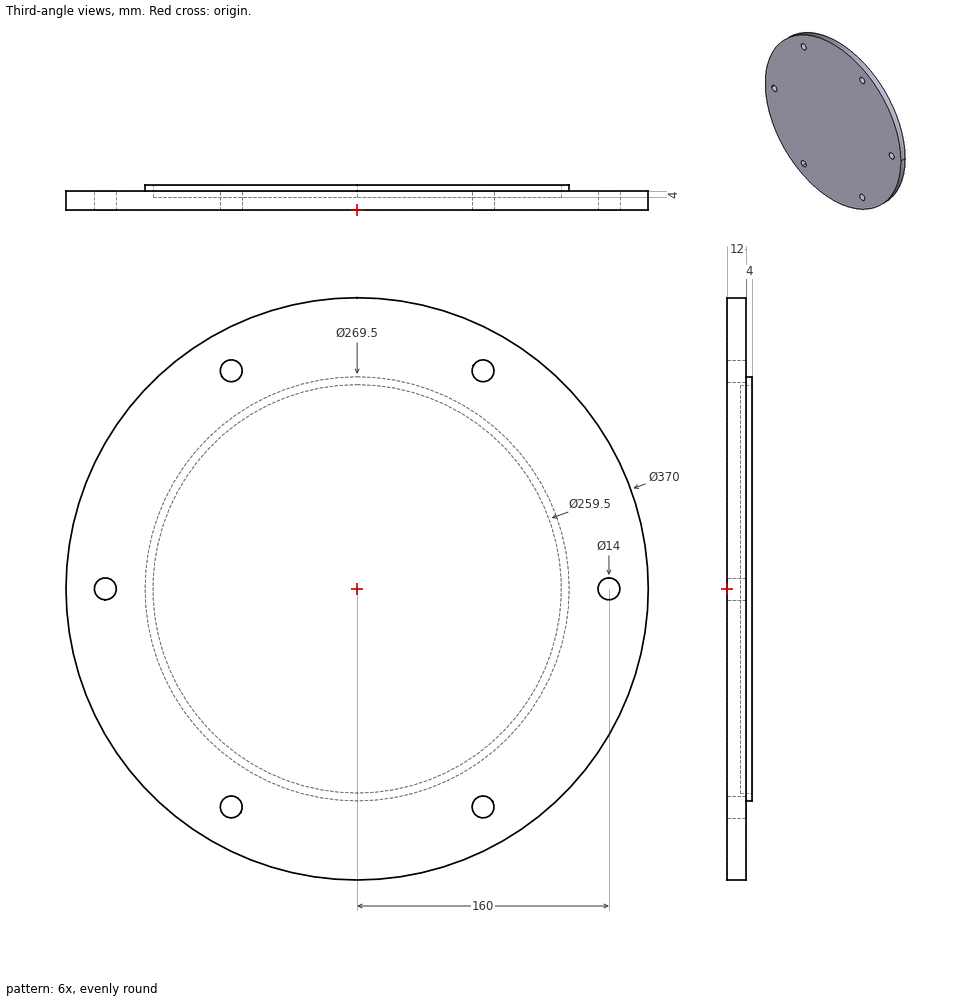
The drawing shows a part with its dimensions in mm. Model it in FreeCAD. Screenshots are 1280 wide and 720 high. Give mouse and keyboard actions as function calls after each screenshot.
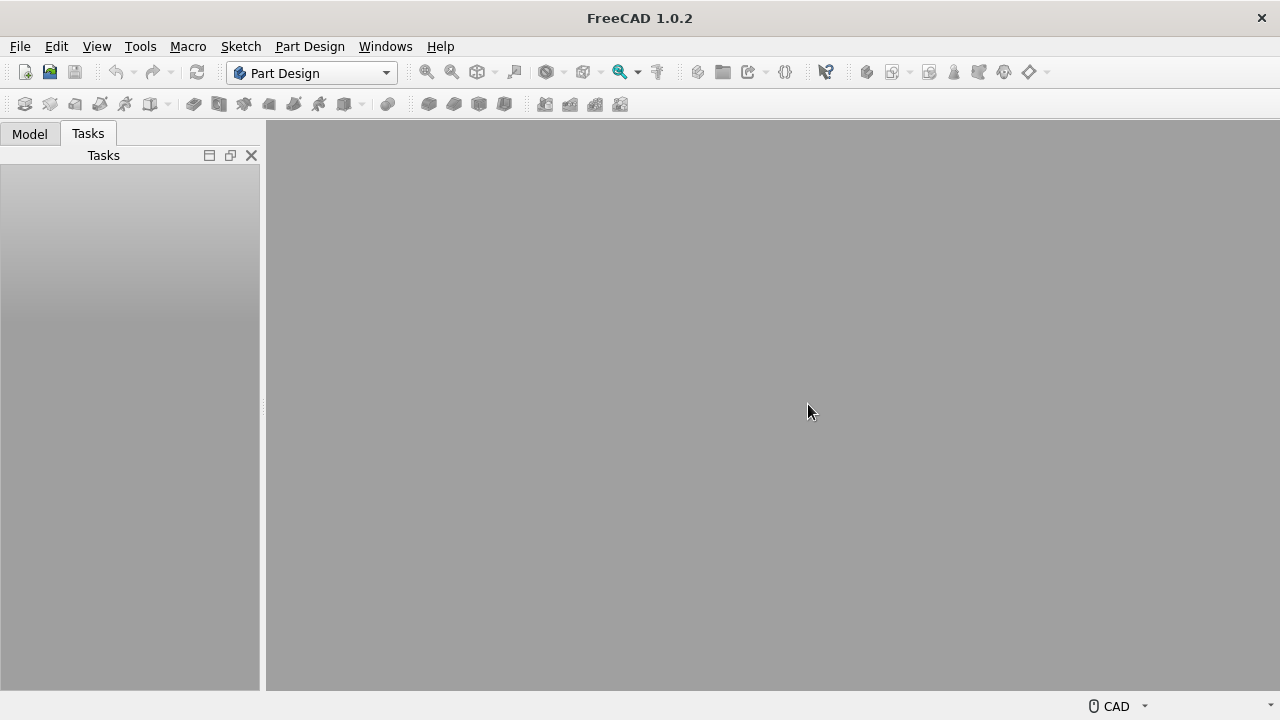
click(25, 72)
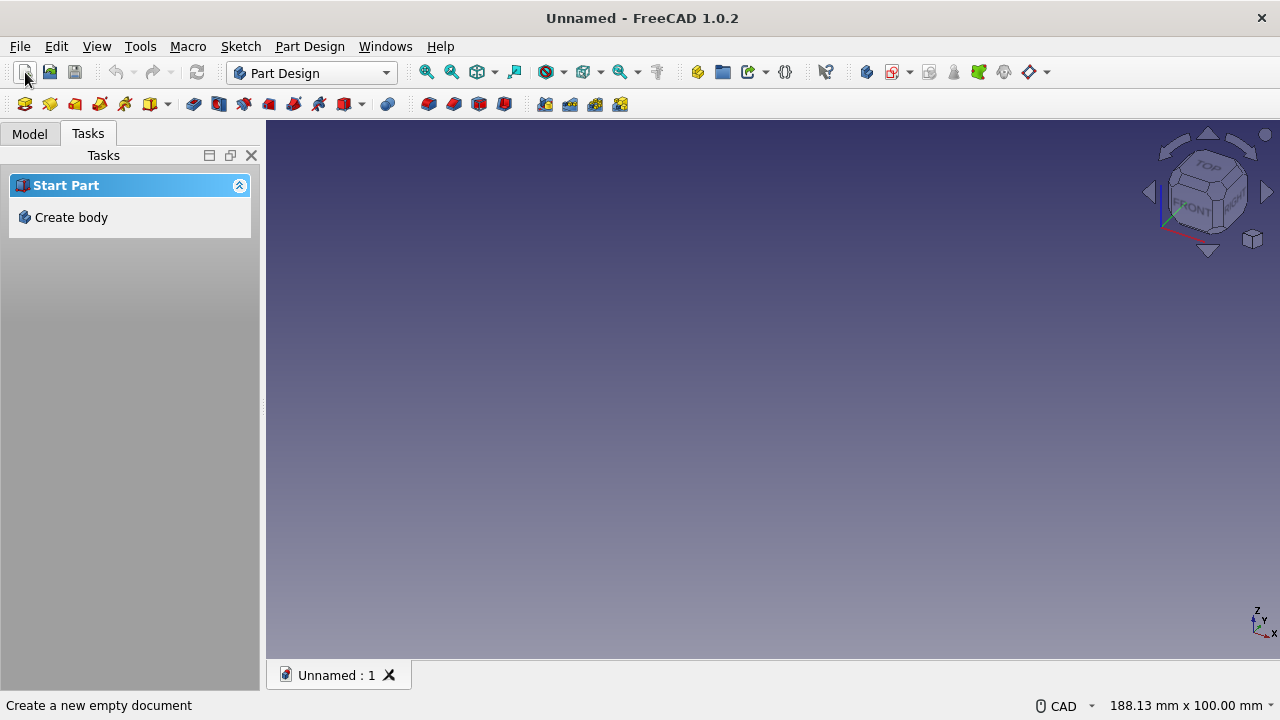
click(892, 72)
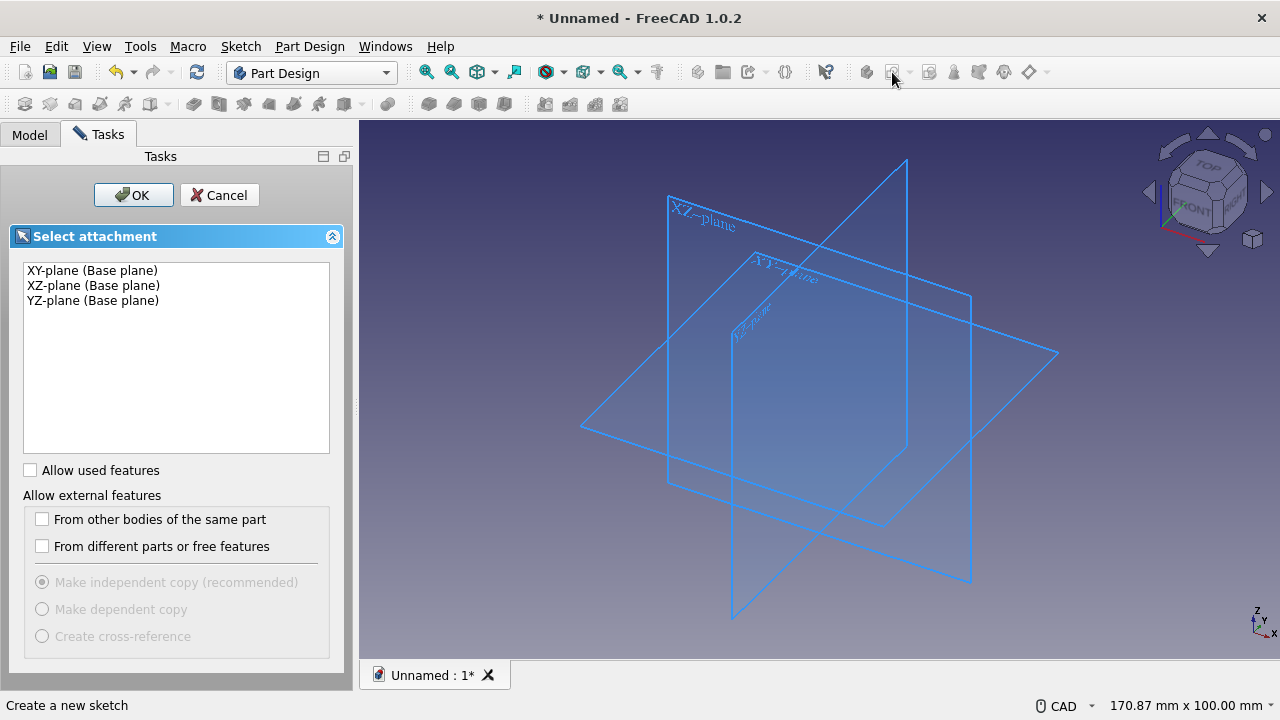
click(84, 286)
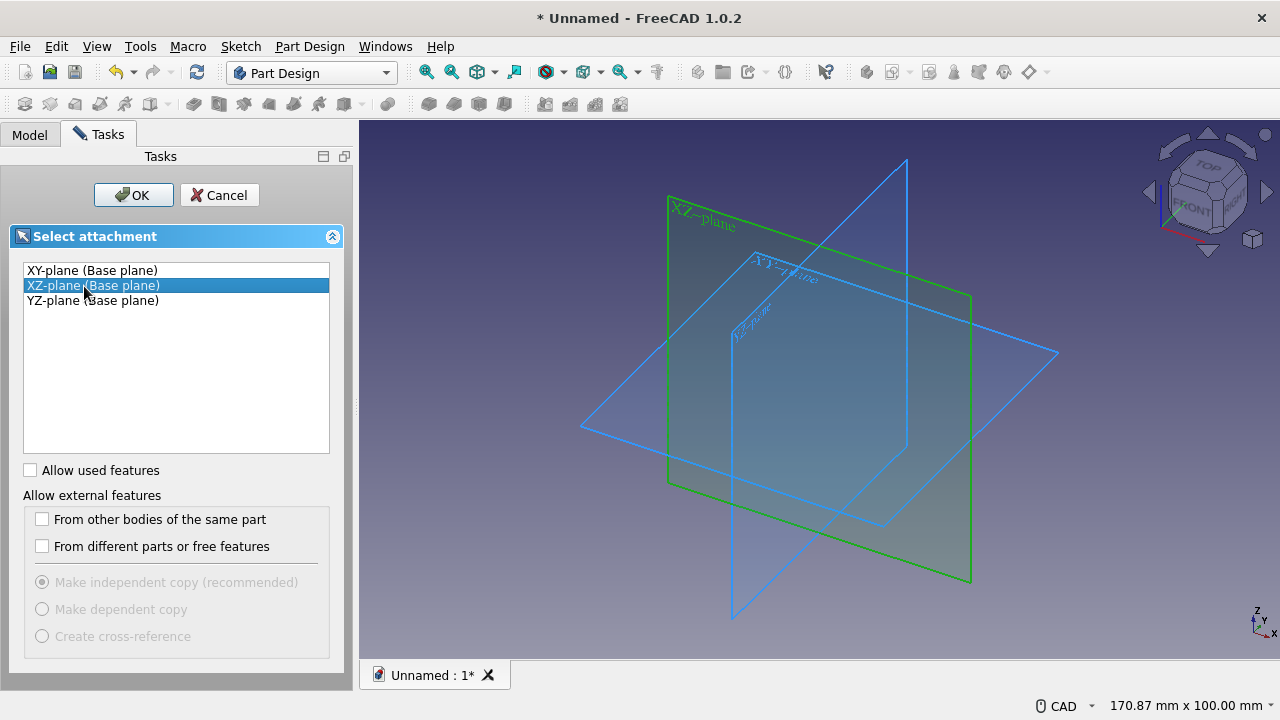
click(134, 195)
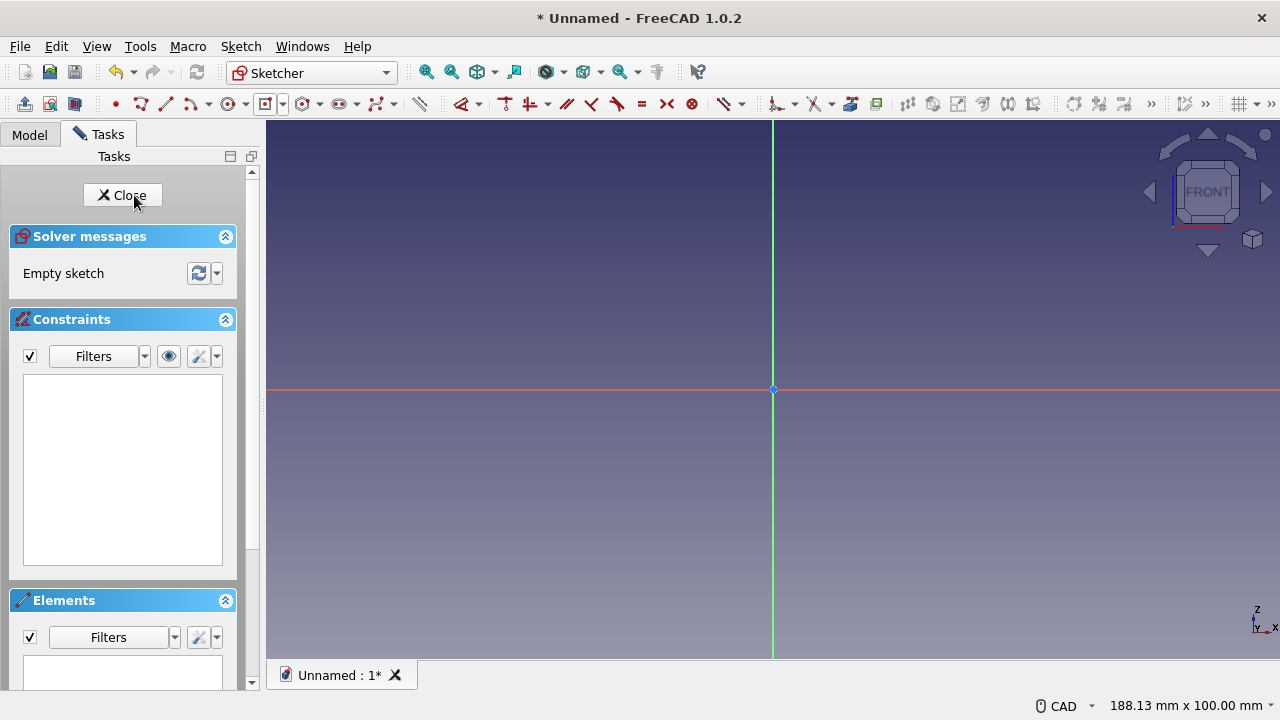
scroll(691, 390, down, 9)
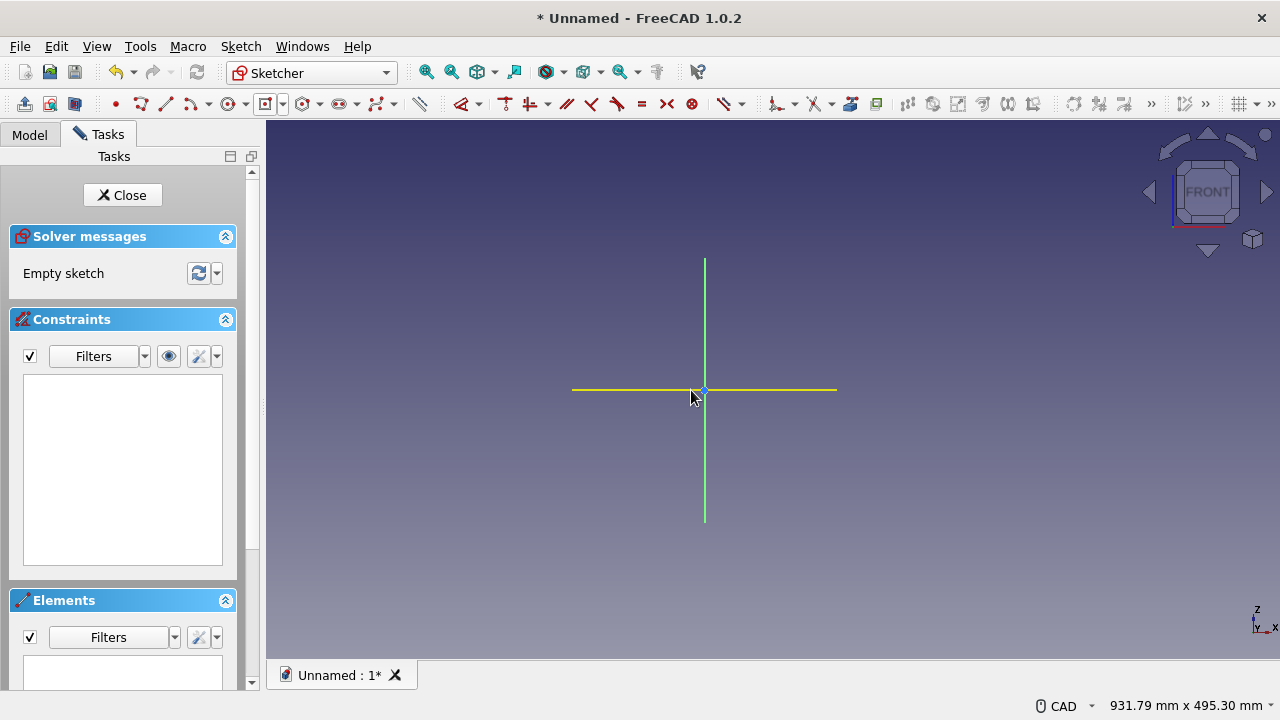
click(228, 104)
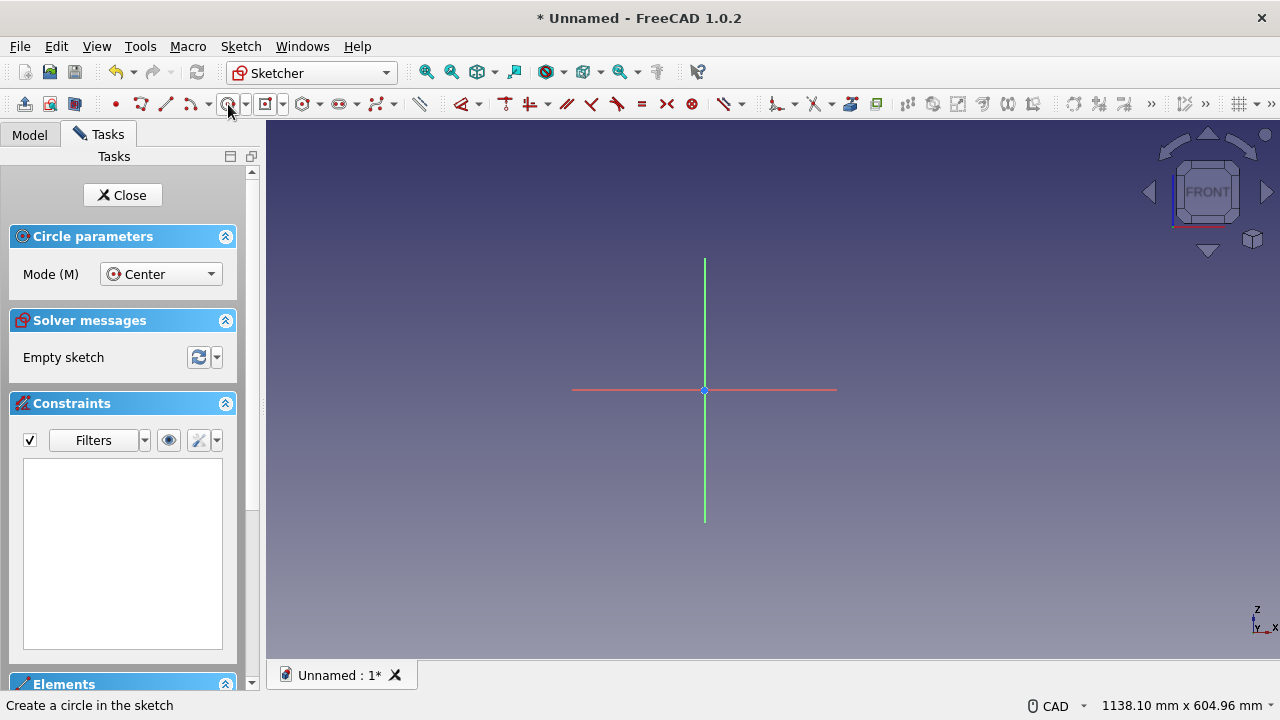
click(705, 390)
click(821, 274)
key(Escape)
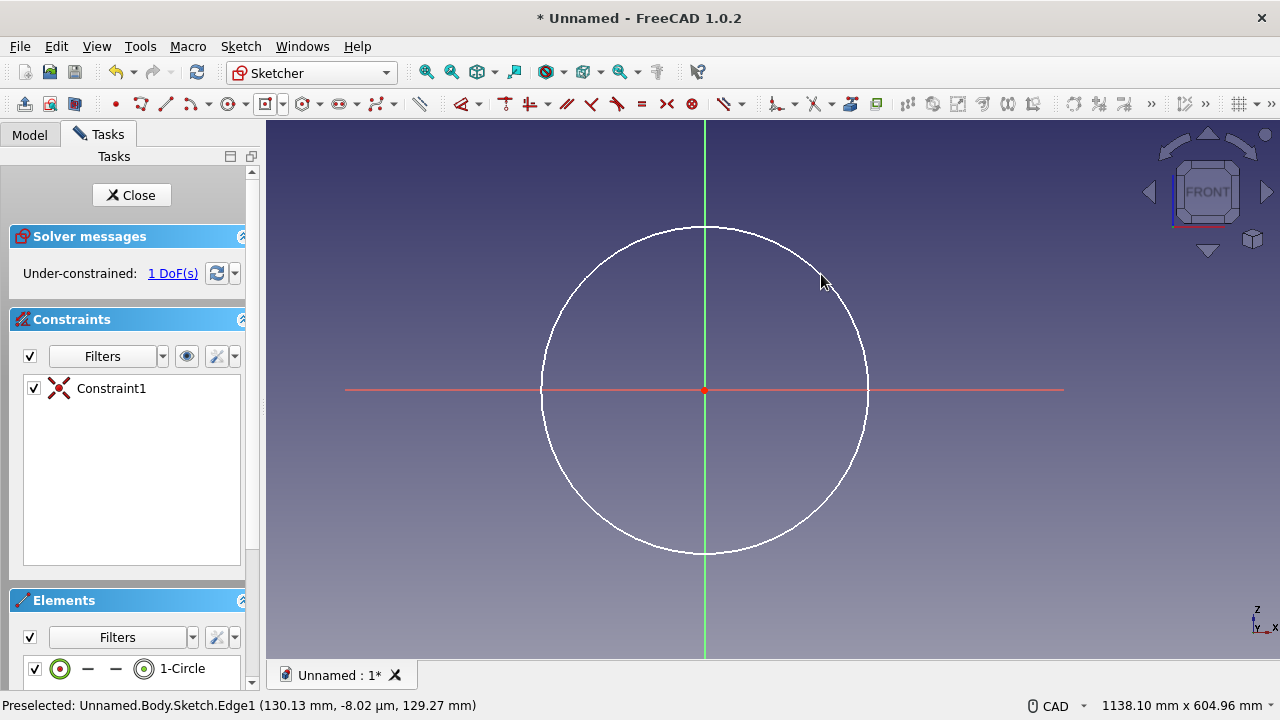
click(460, 104)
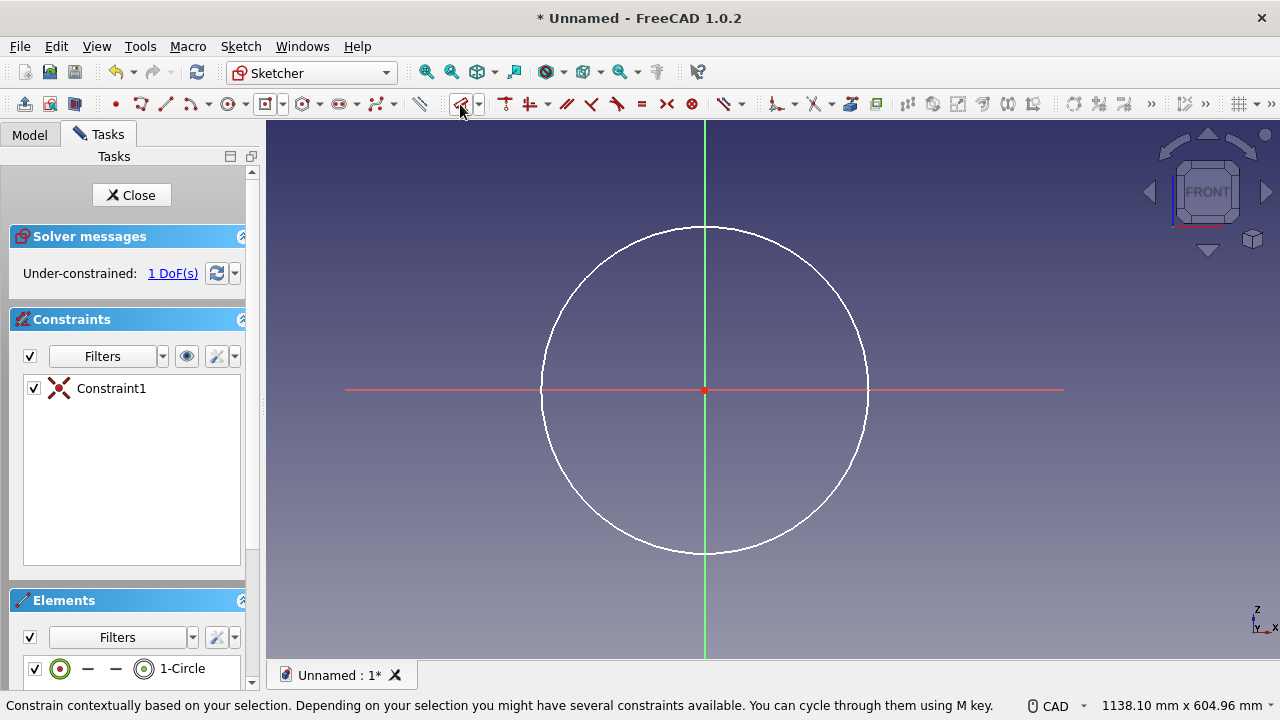
click(820, 274)
click(843, 251)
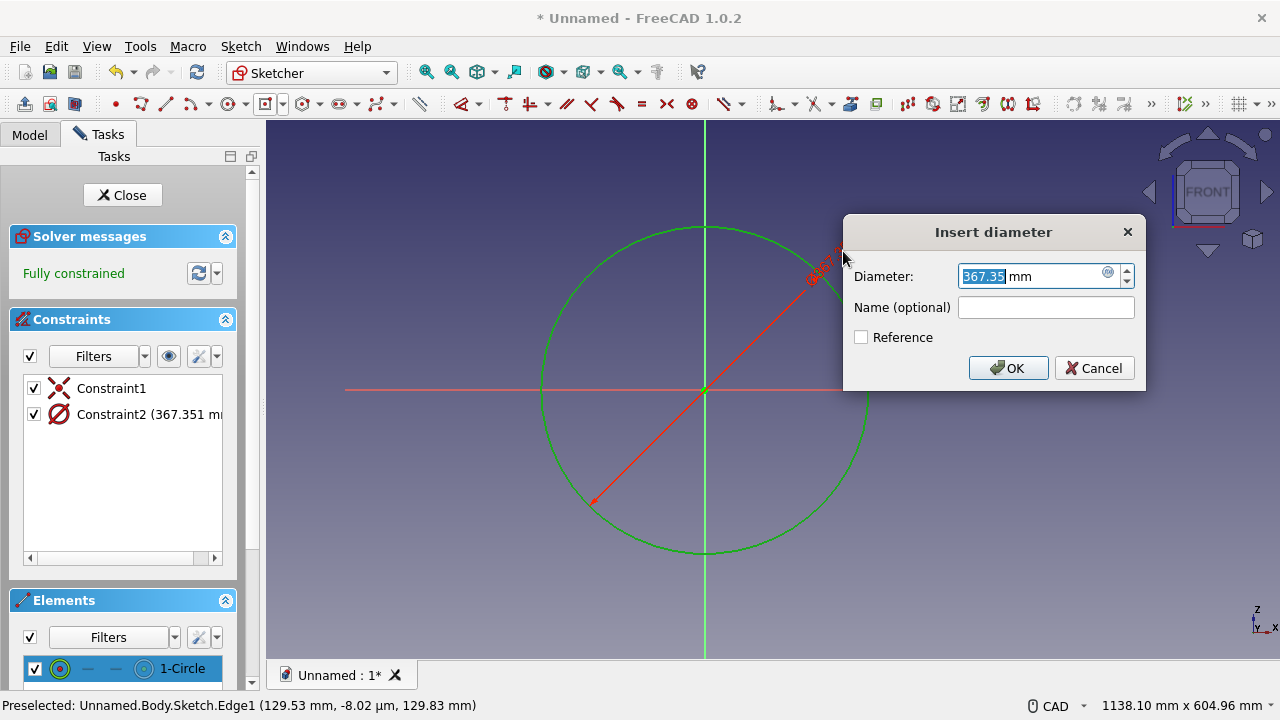
text(370)
key(Return)
key(Escape)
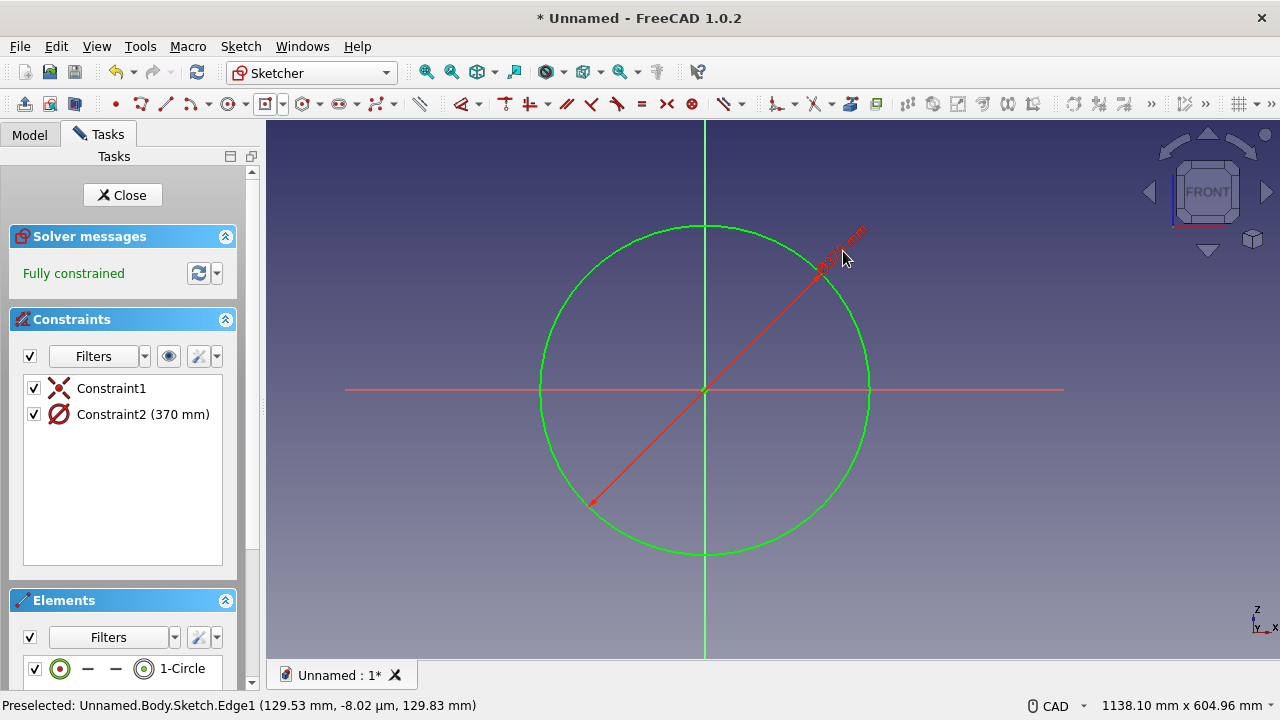
click(123, 195)